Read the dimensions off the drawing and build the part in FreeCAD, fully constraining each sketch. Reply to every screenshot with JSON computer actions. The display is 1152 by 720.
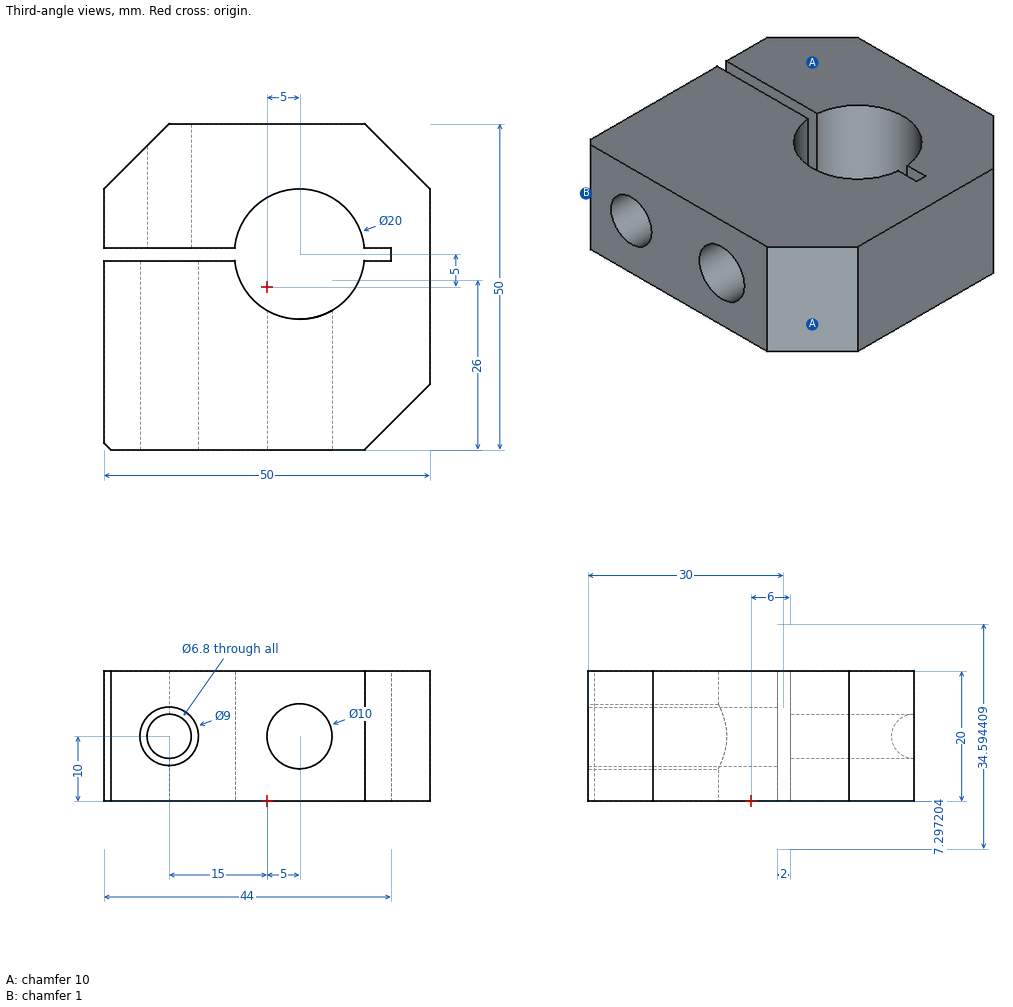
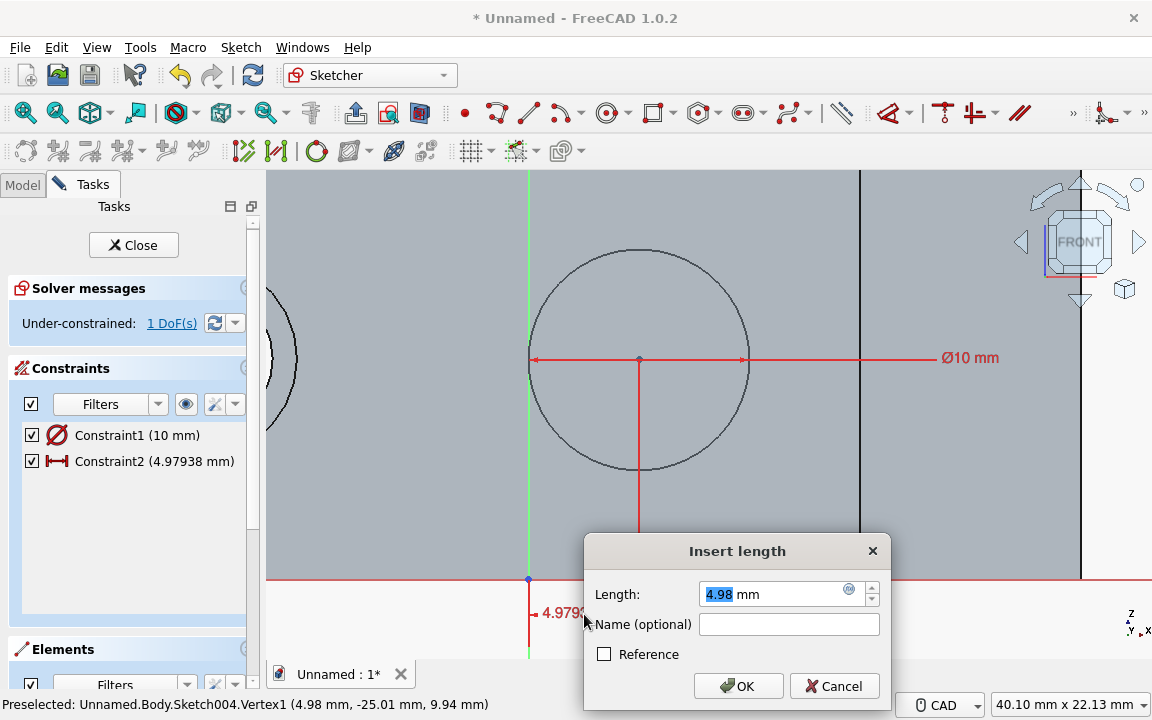
{"action": "type", "text": "5"}
{"action": "key", "text": "Return"}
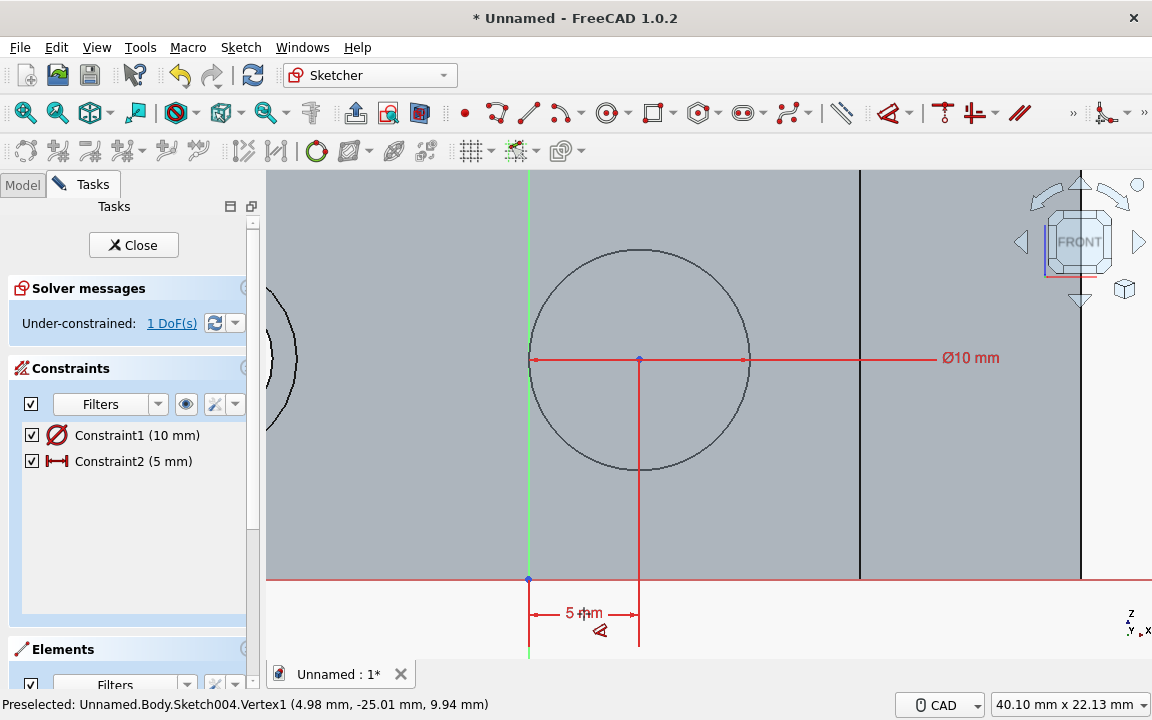
{"action": "left_click", "coordinate": [639, 360]}
{"action": "left_click", "coordinate": [495, 470]}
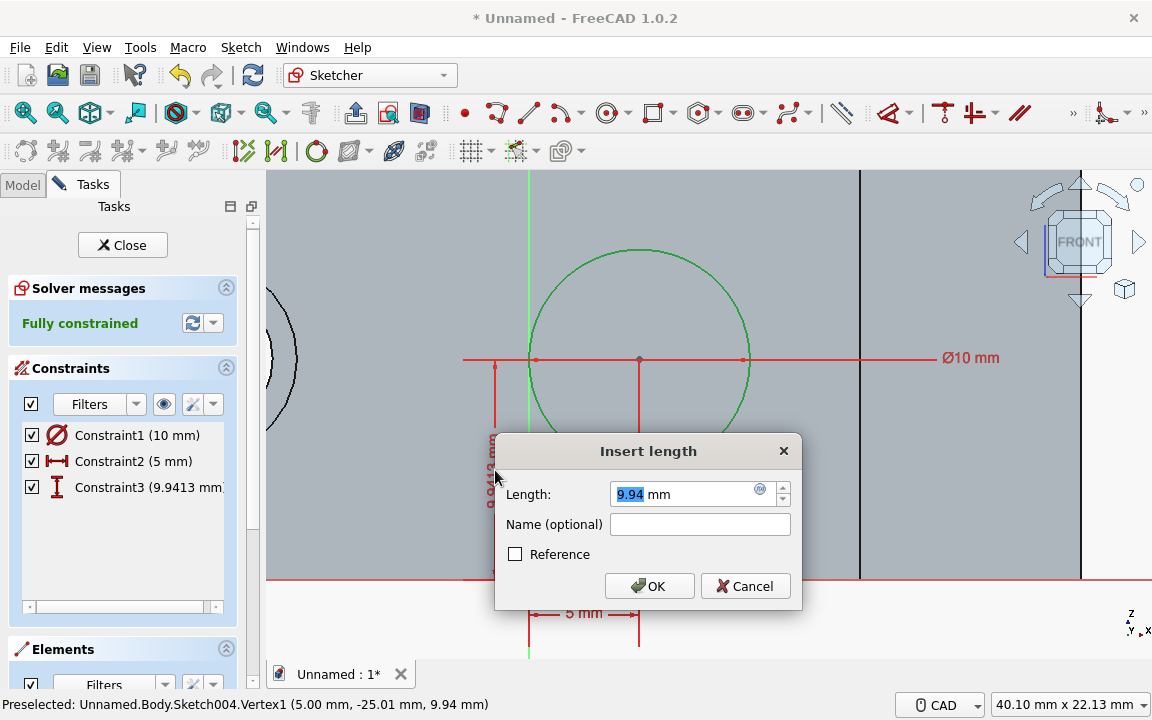
{"action": "type", "text": "10"}
{"action": "key", "text": "Return"}
{"action": "key", "text": "Escape"}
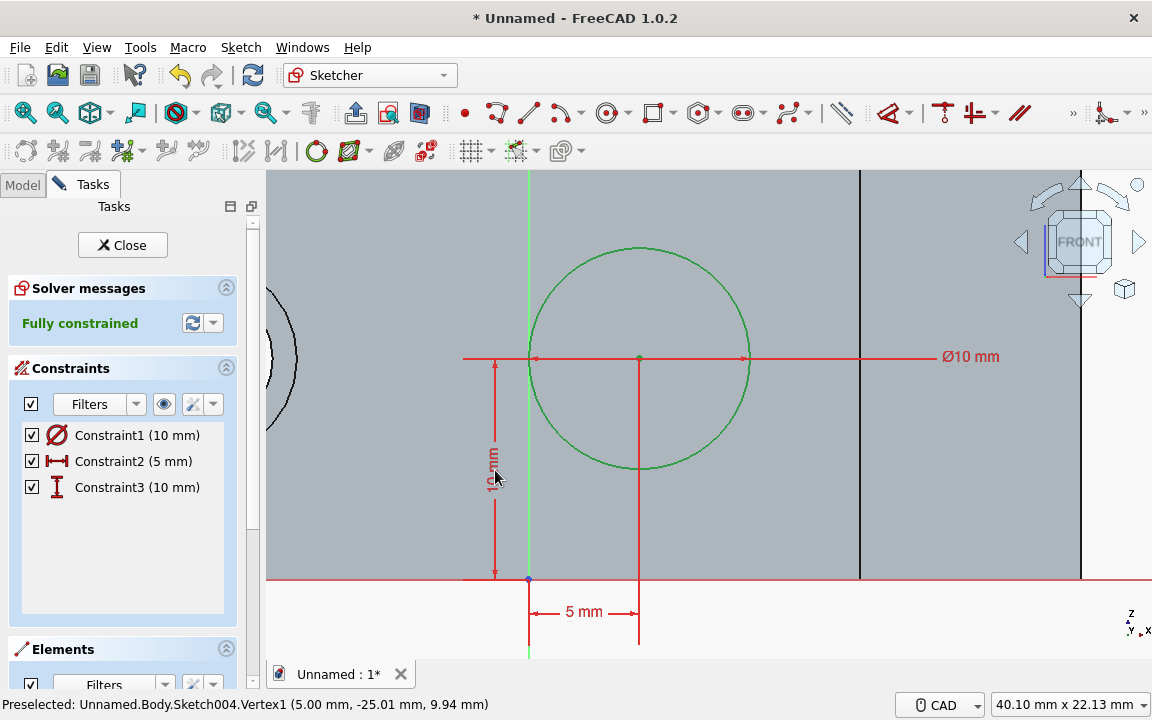
{"action": "left_click", "coordinate": [123, 245]}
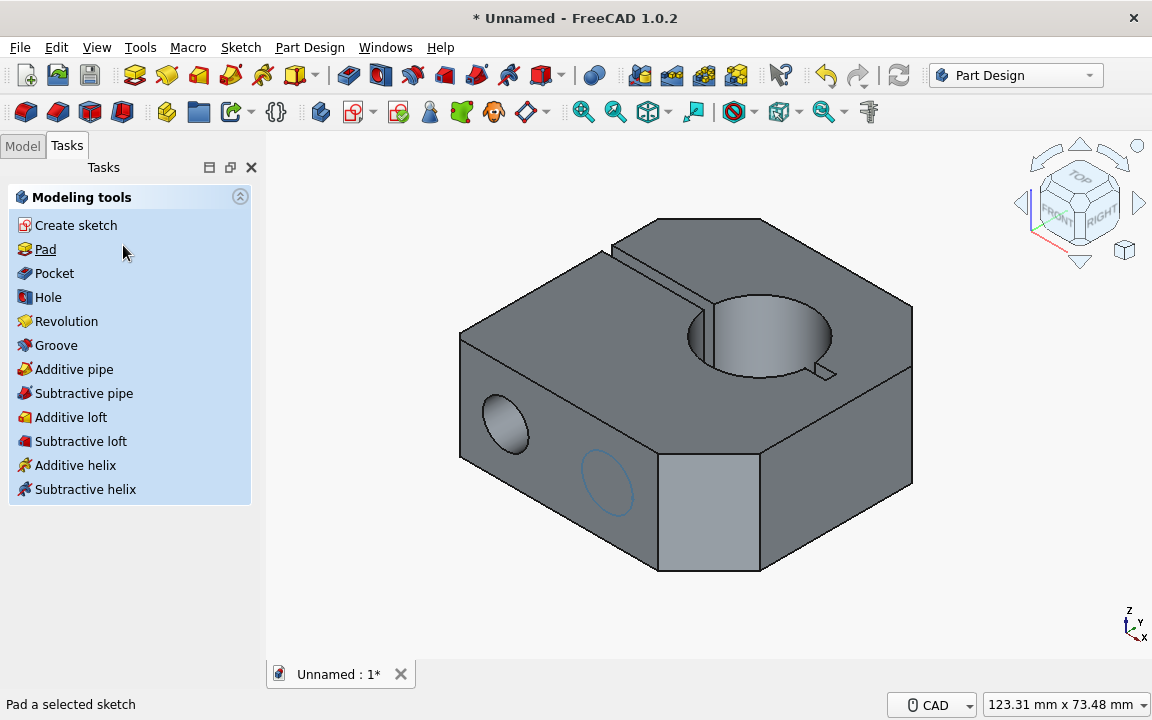
{"action": "left_click", "coordinate": [350, 76]}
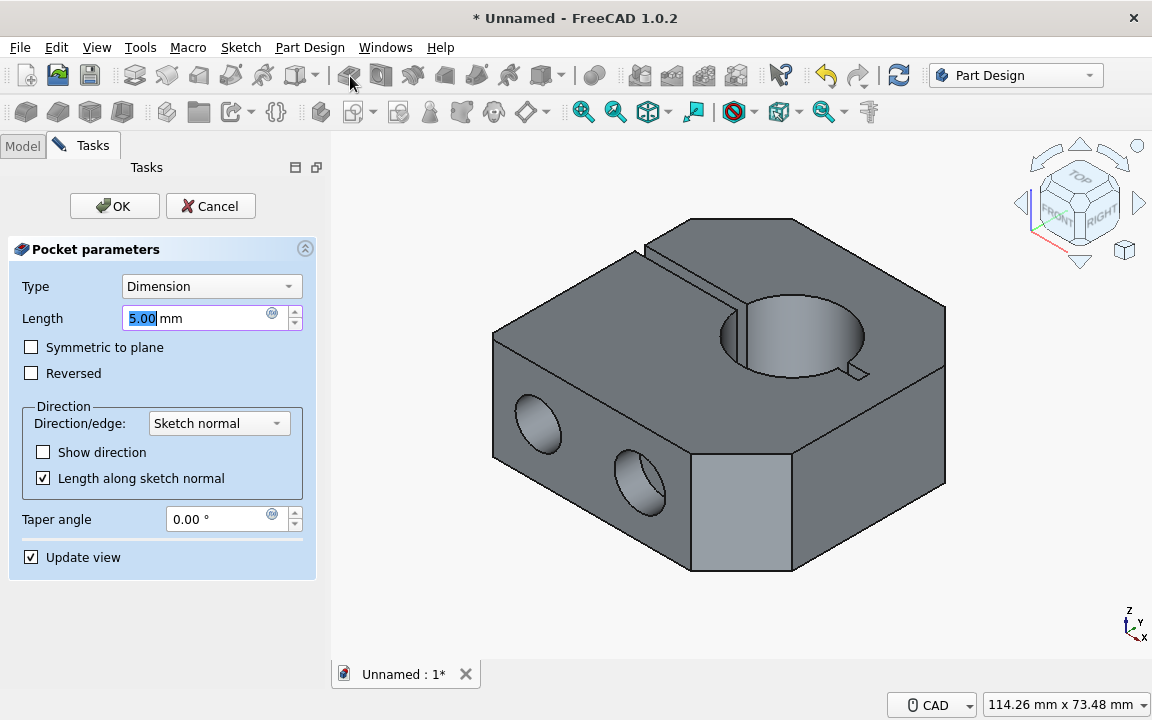
{"action": "type", "text": "26"}
{"action": "key", "text": "Tab"}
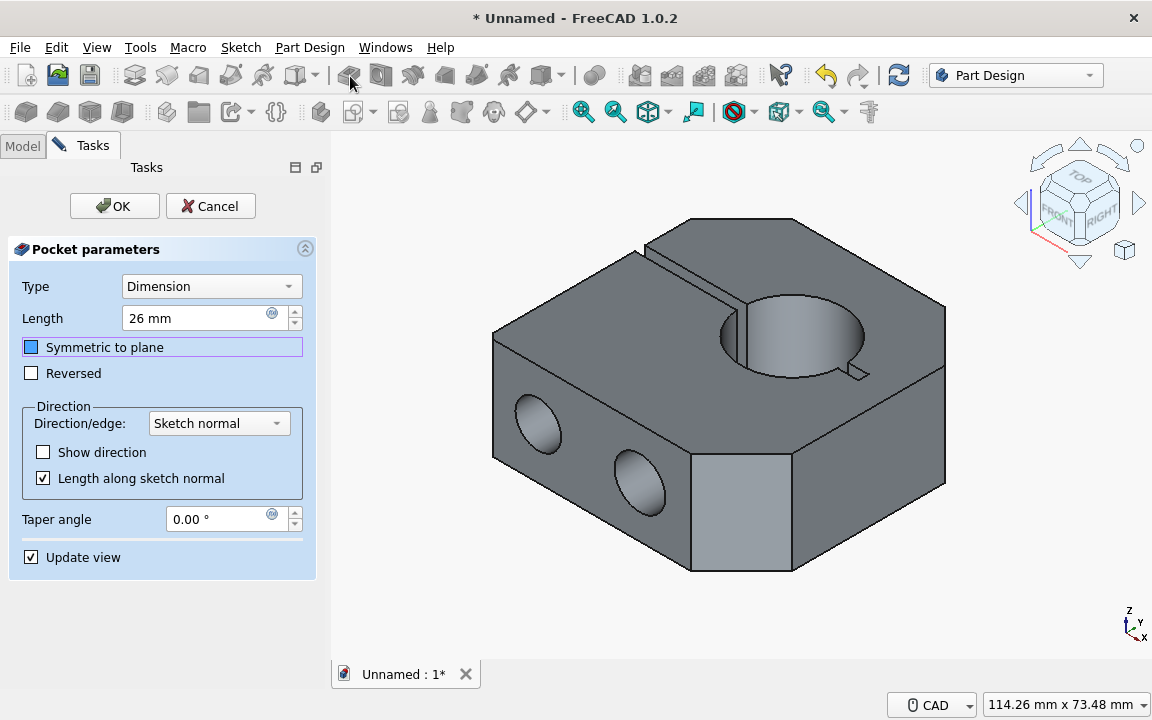
{"action": "left_click", "coordinate": [115, 206]}